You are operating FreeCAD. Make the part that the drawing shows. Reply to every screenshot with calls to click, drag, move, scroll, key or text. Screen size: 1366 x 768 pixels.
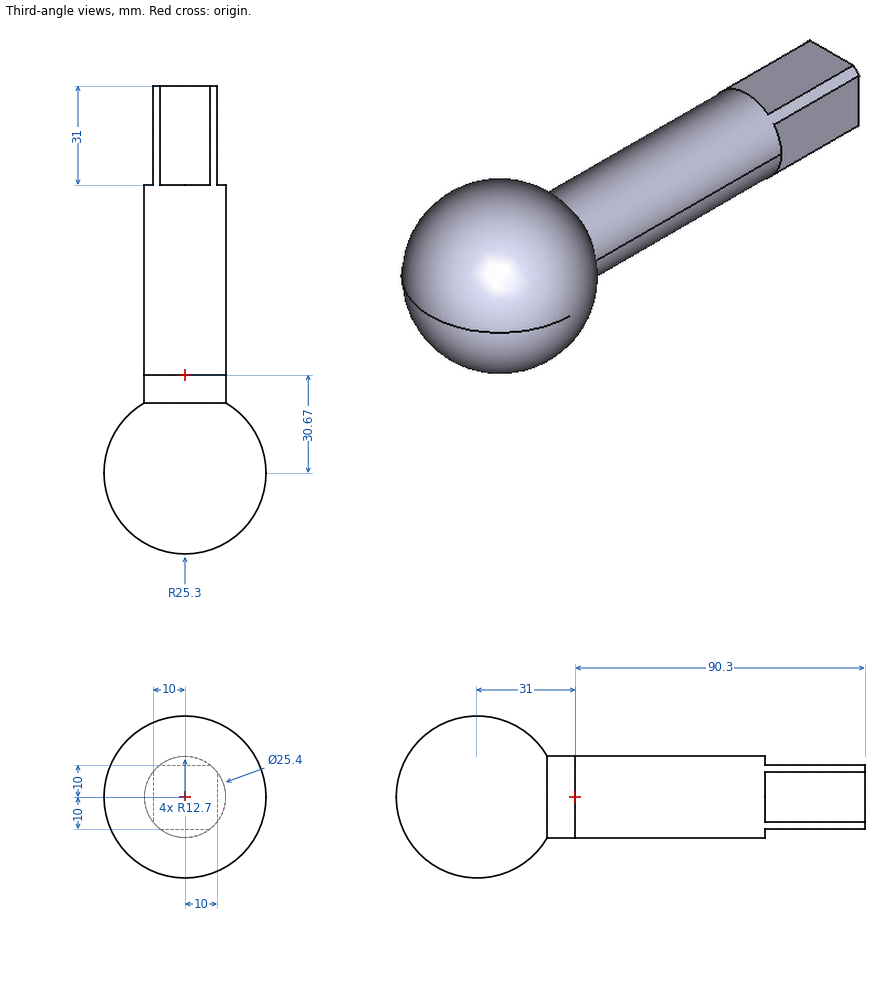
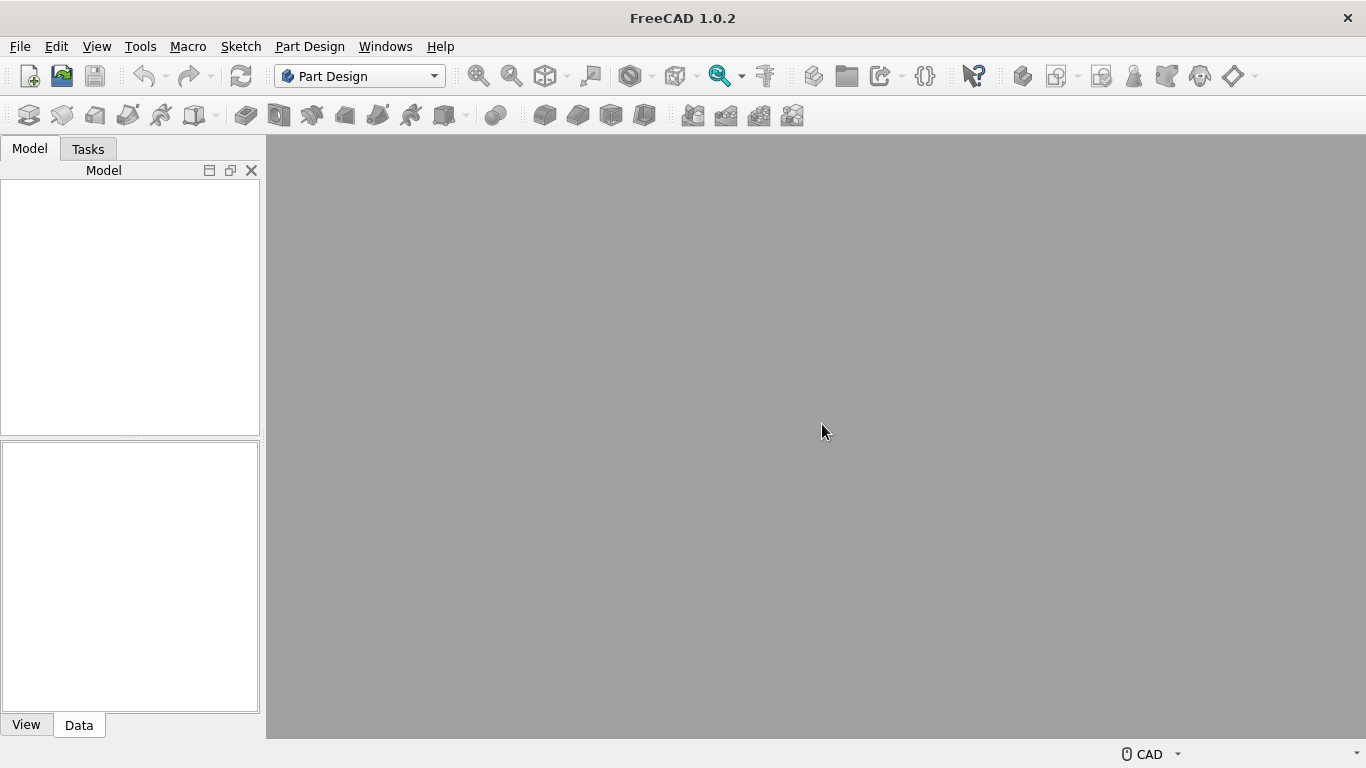
click(29, 76)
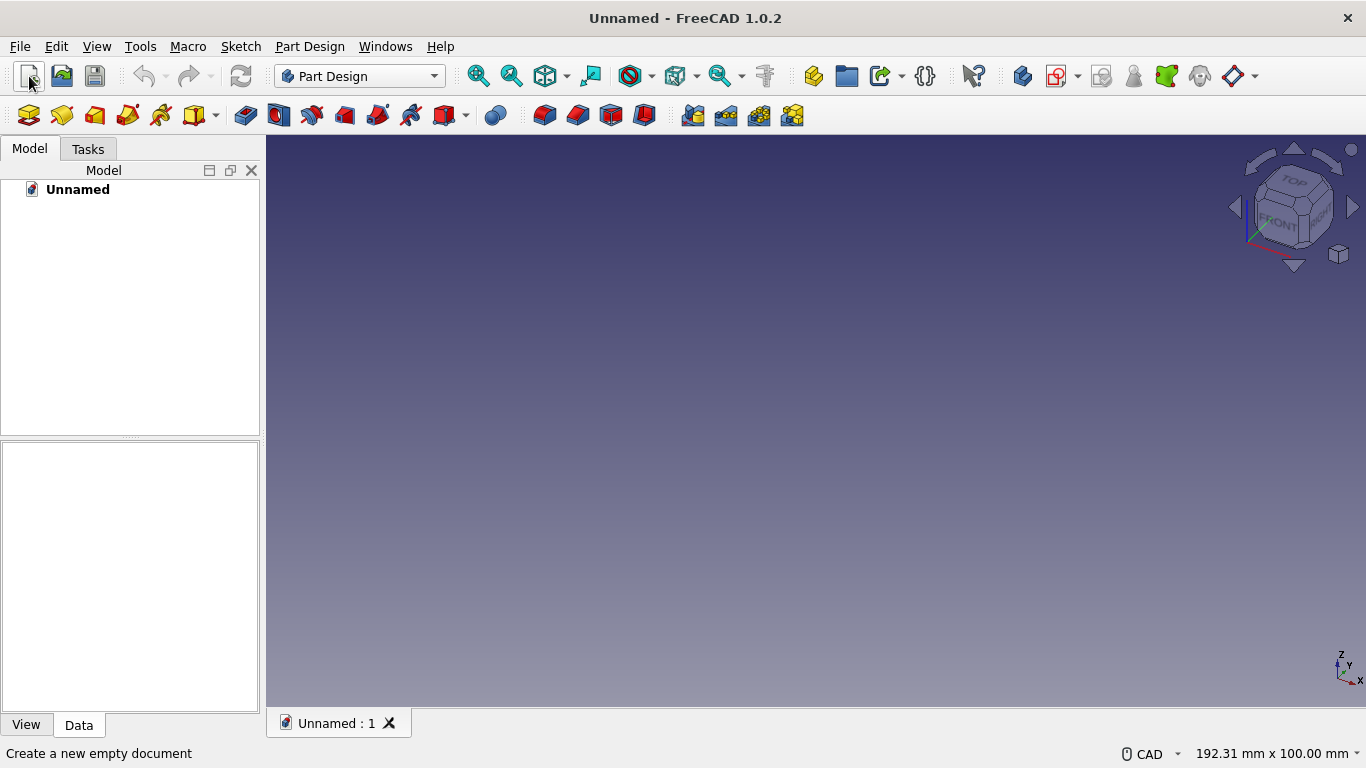
click(1056, 76)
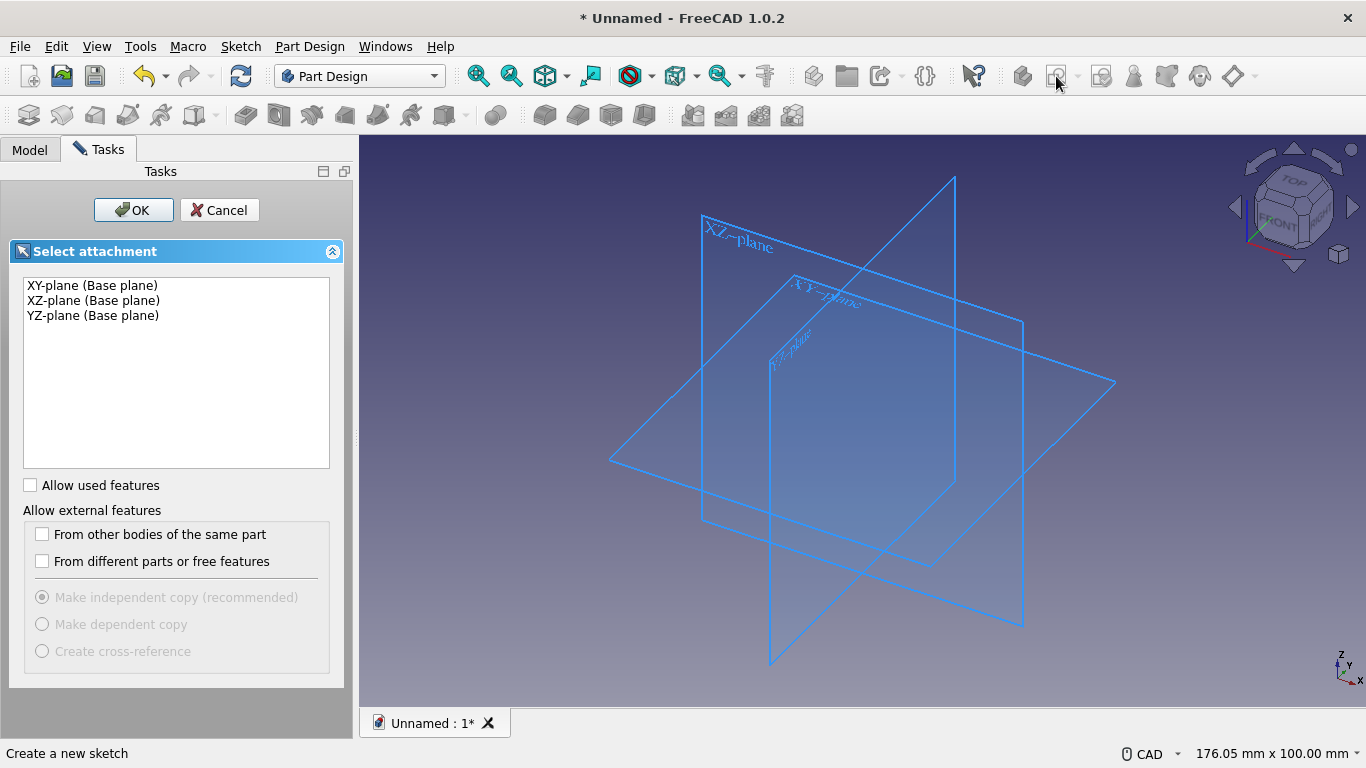
click(84, 300)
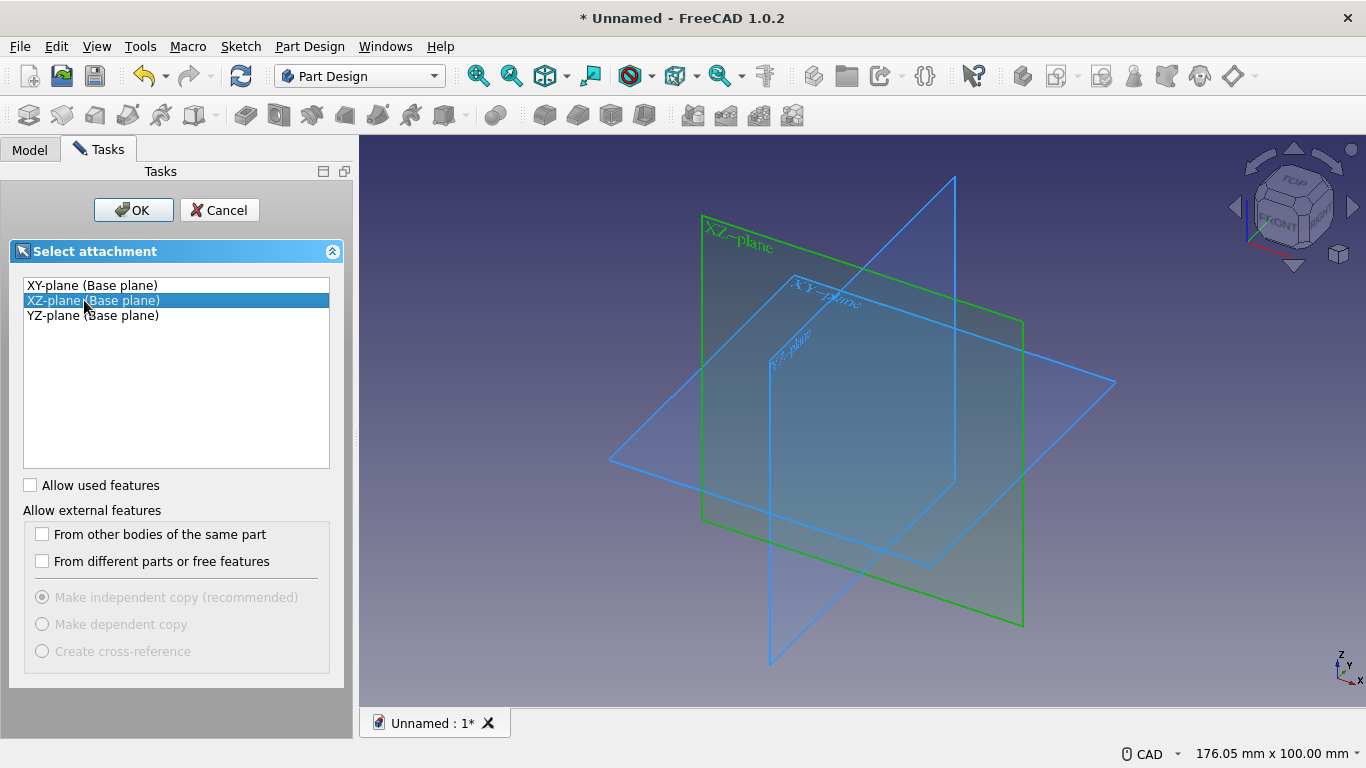
click(134, 210)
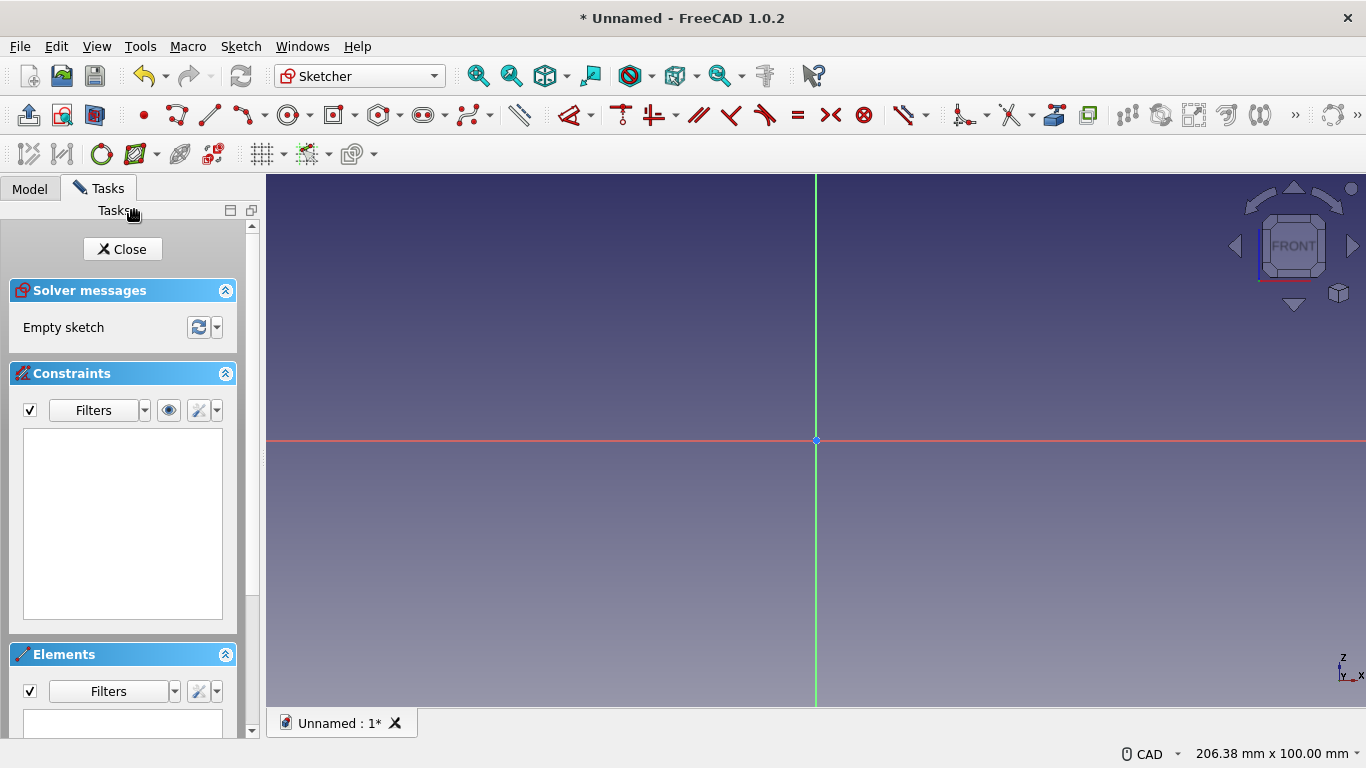
scroll(856, 440, up, 5)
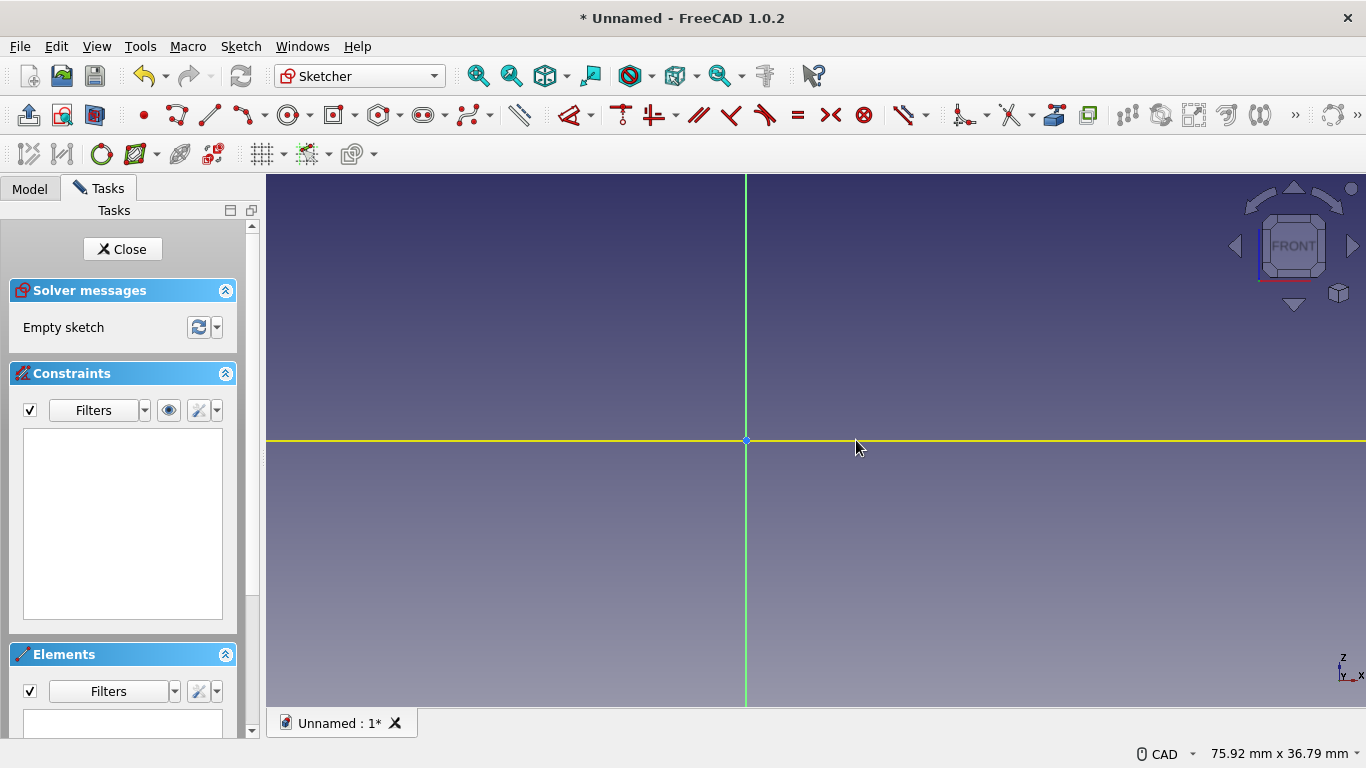
click(288, 116)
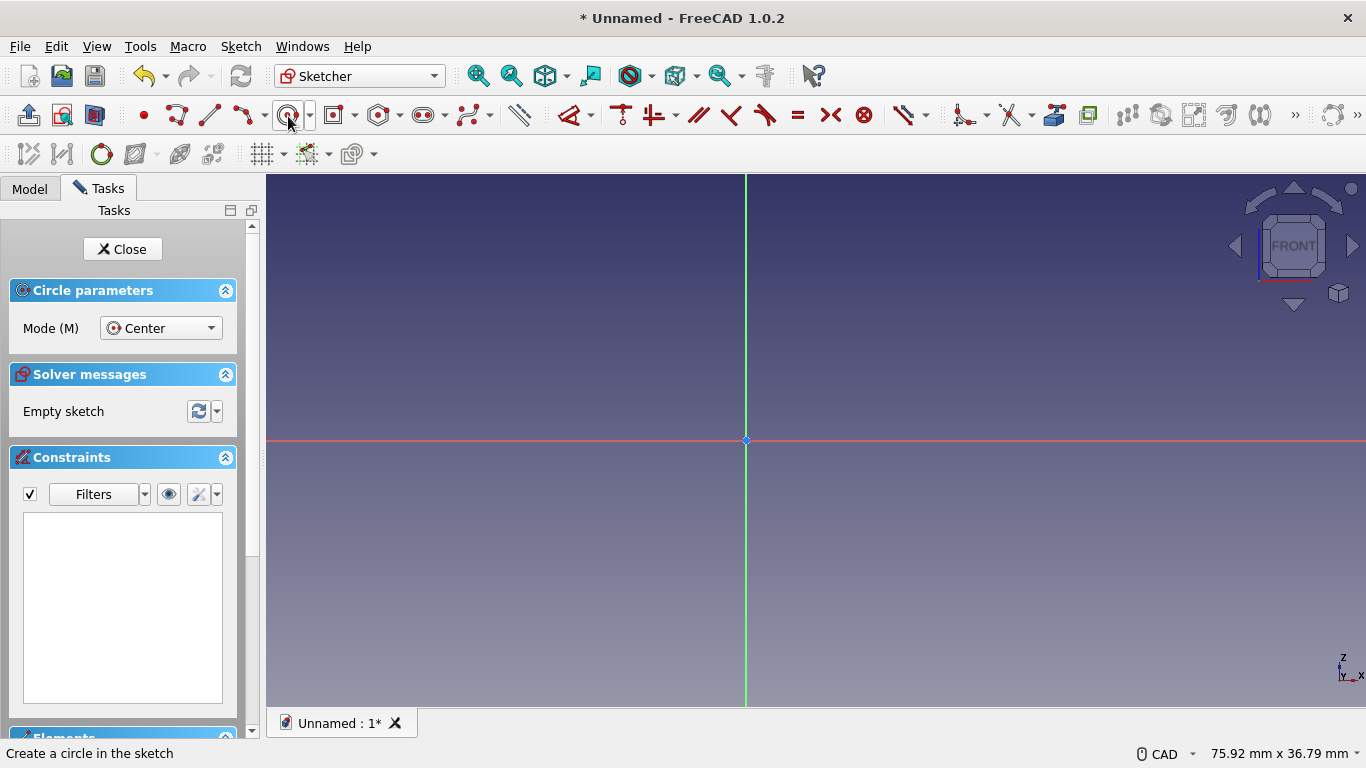
click(746, 440)
move(876, 310)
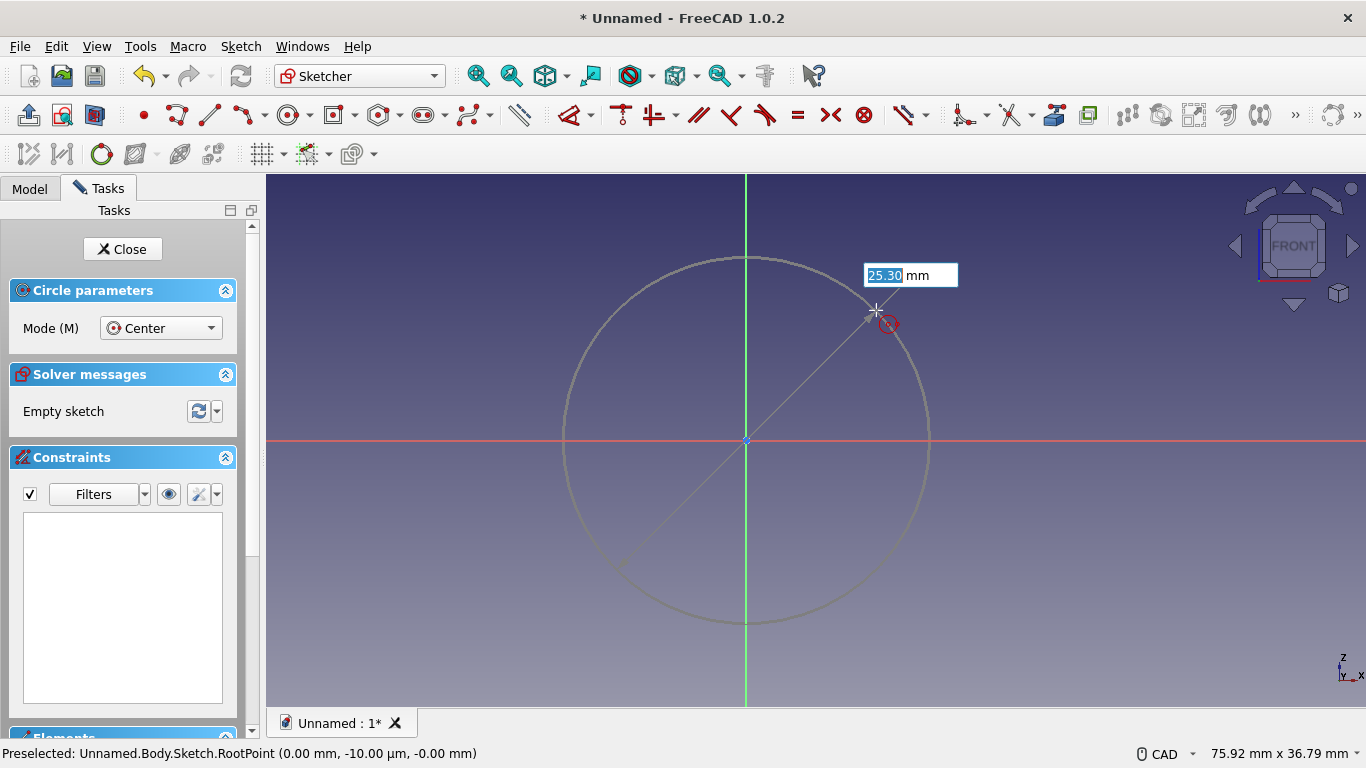
text(25.4)
key(Return)
key(Escape)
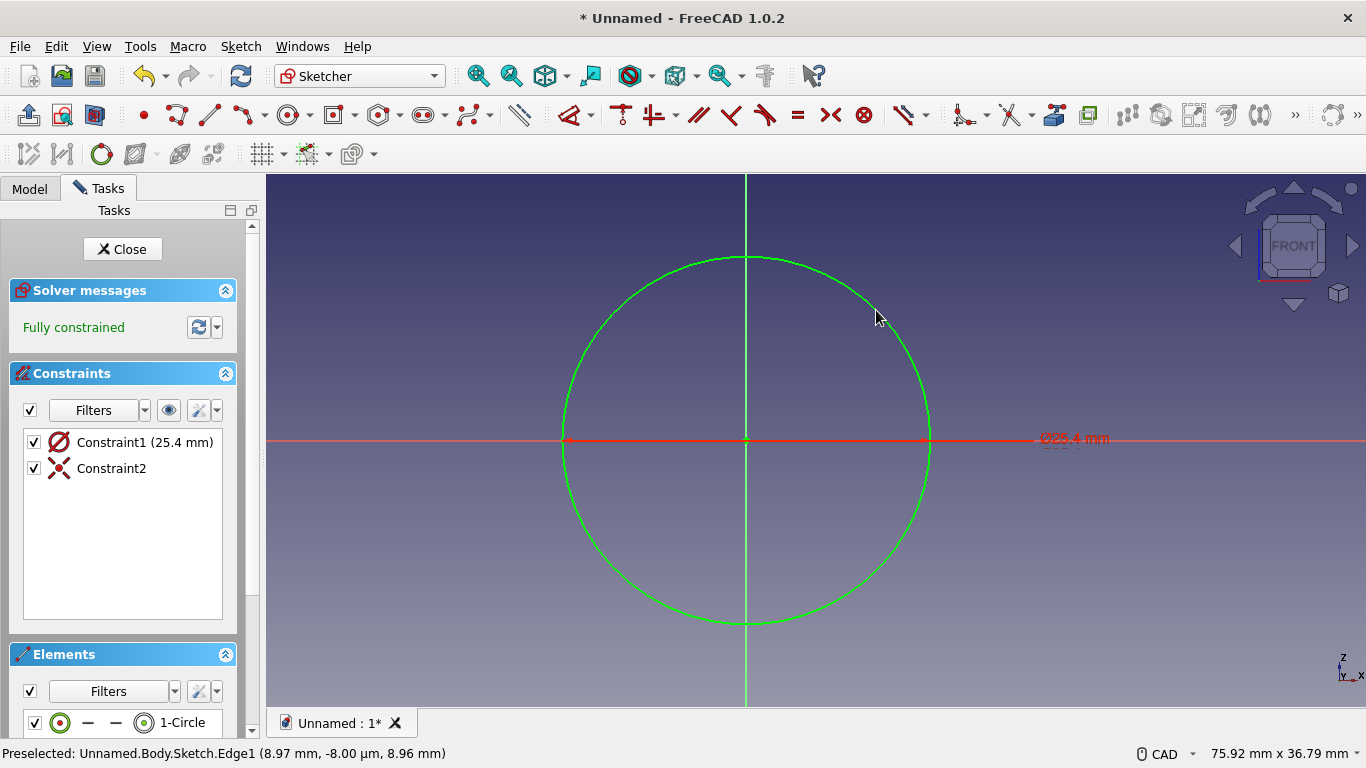
click(123, 249)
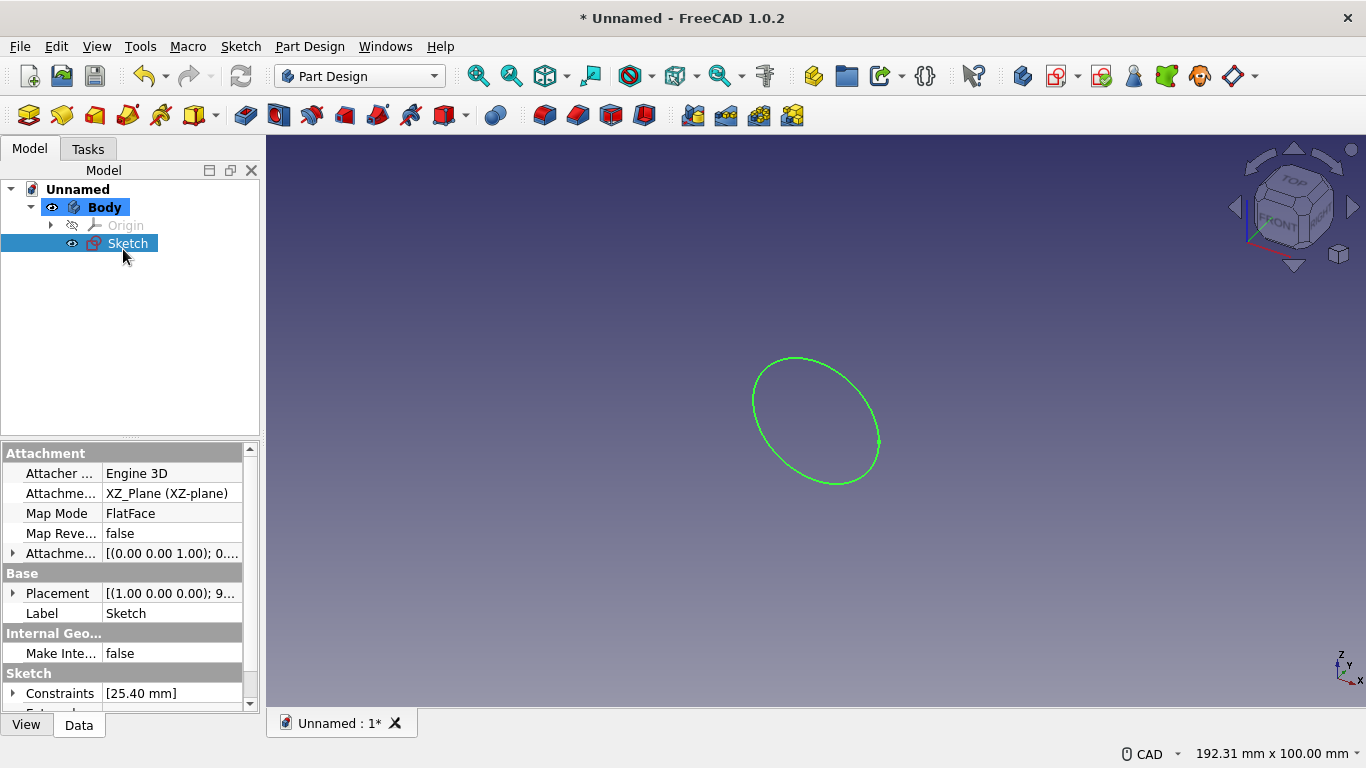
click(29, 116)